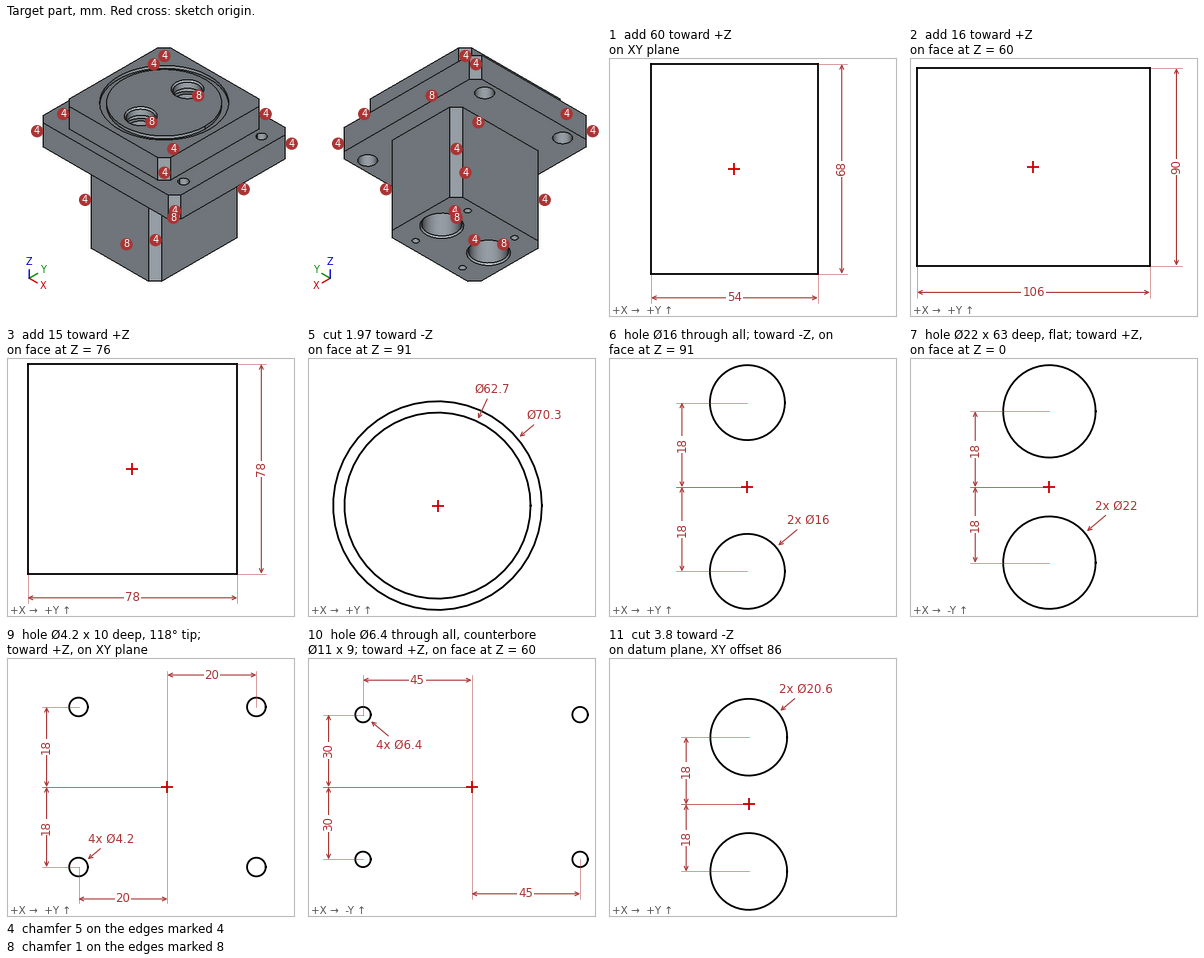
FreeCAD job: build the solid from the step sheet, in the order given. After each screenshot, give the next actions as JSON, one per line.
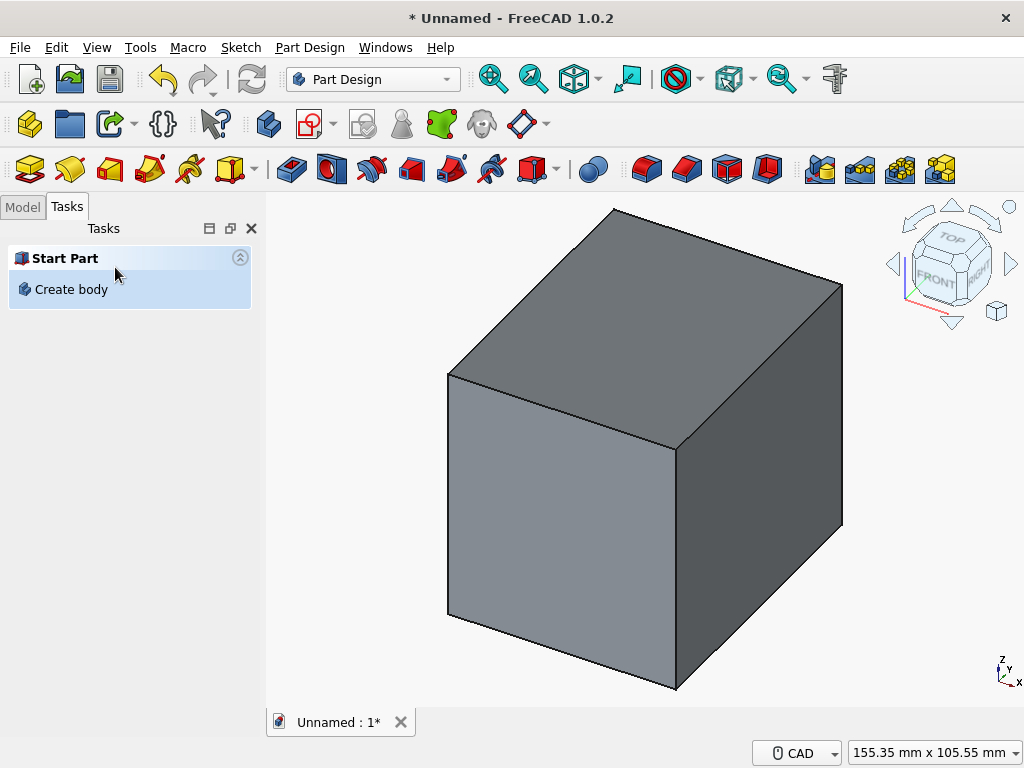
{"action": "left_click", "coordinate": [645, 329]}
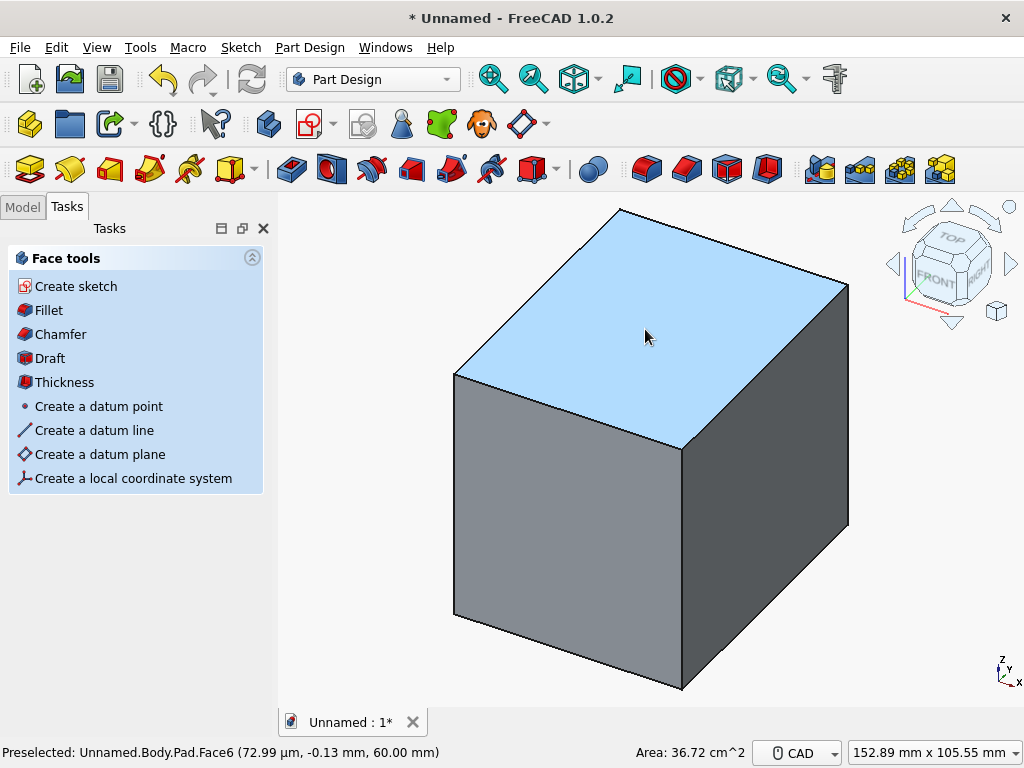
{"action": "left_click", "coordinate": [310, 124]}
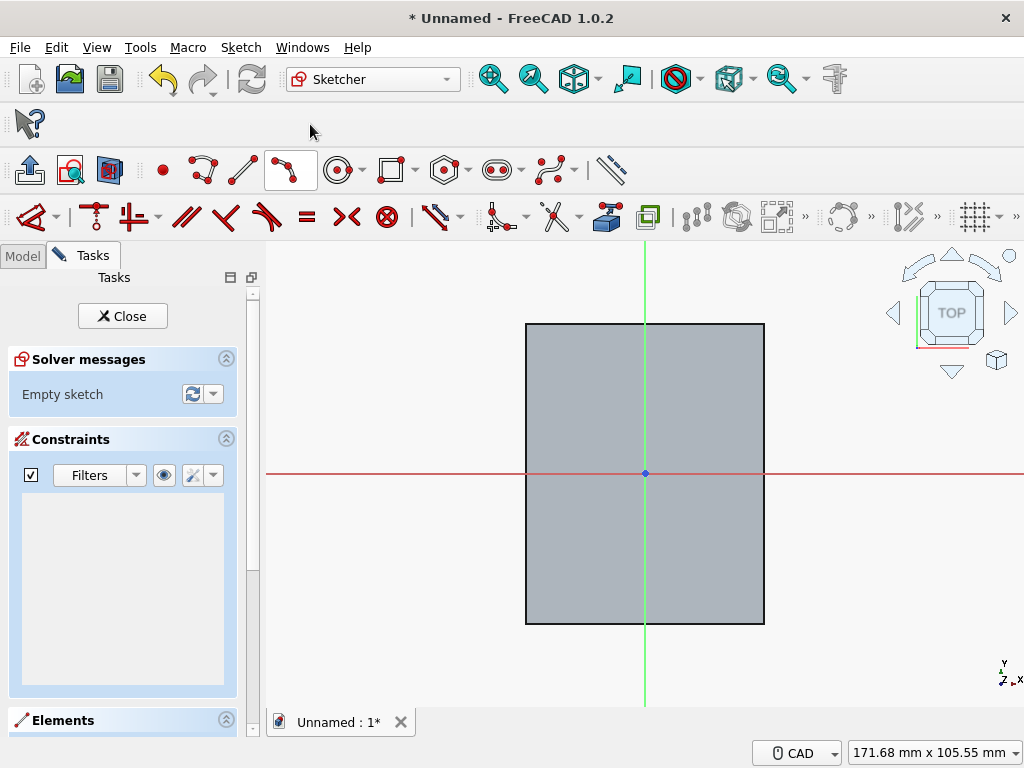
{"action": "scroll", "coordinate": [437, 474], "scroll_direction": "down", "scroll_amount": 2}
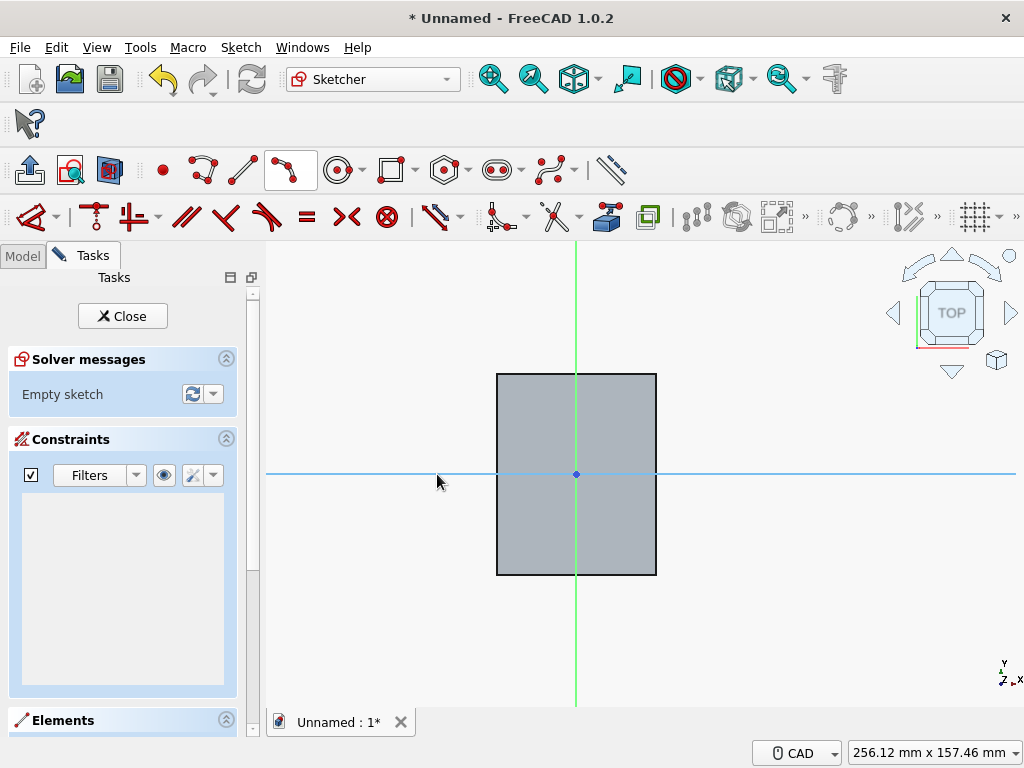
{"action": "key", "text": "g v"}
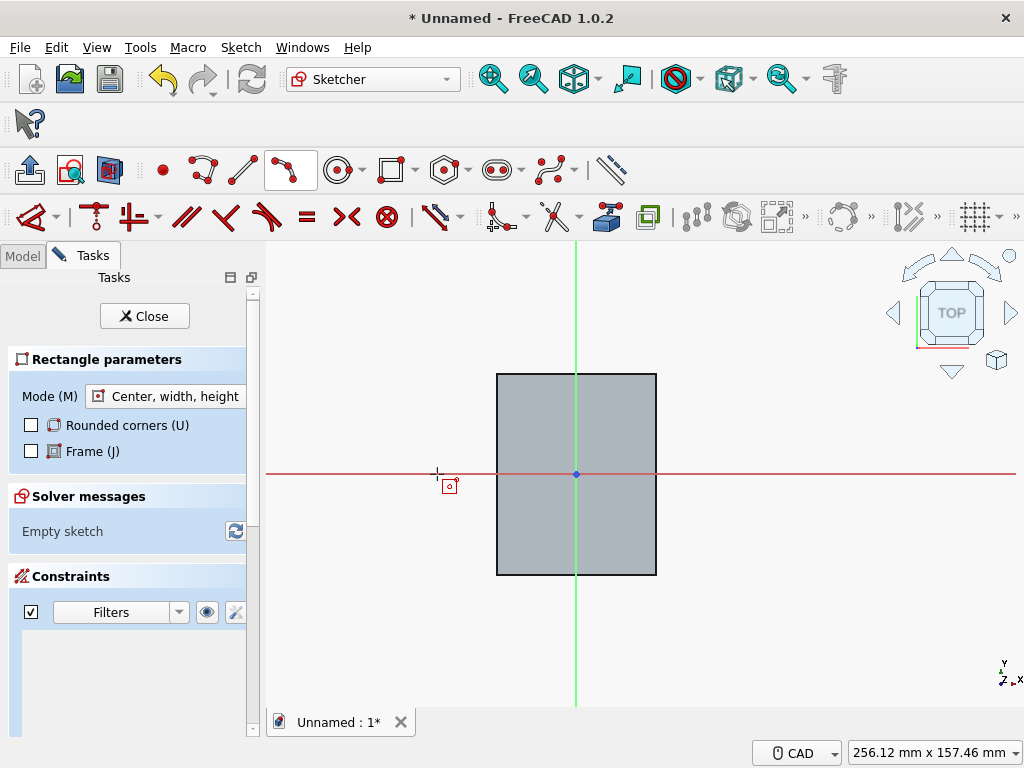
{"action": "left_click", "coordinate": [577, 474]}
{"action": "mouse_move", "coordinate": [733, 341]}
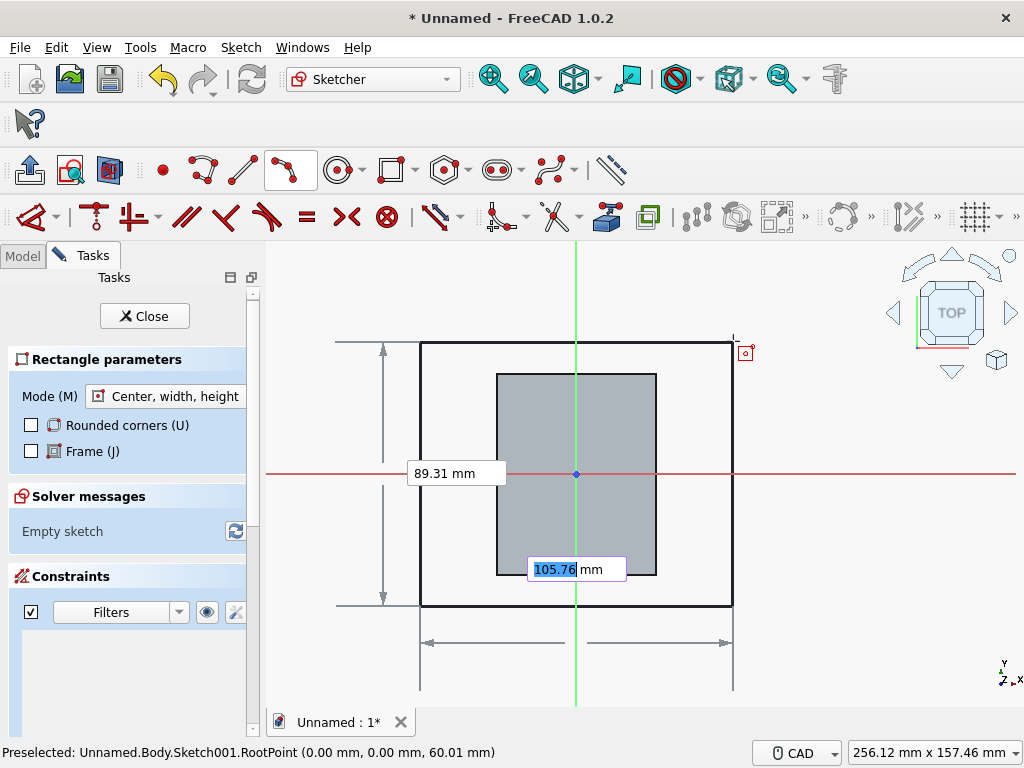
{"action": "type", "text": "106"}
{"action": "key", "text": "Tab"}
{"action": "type", "text": "90"}
{"action": "key", "text": "Return"}
{"action": "key", "text": "Escape"}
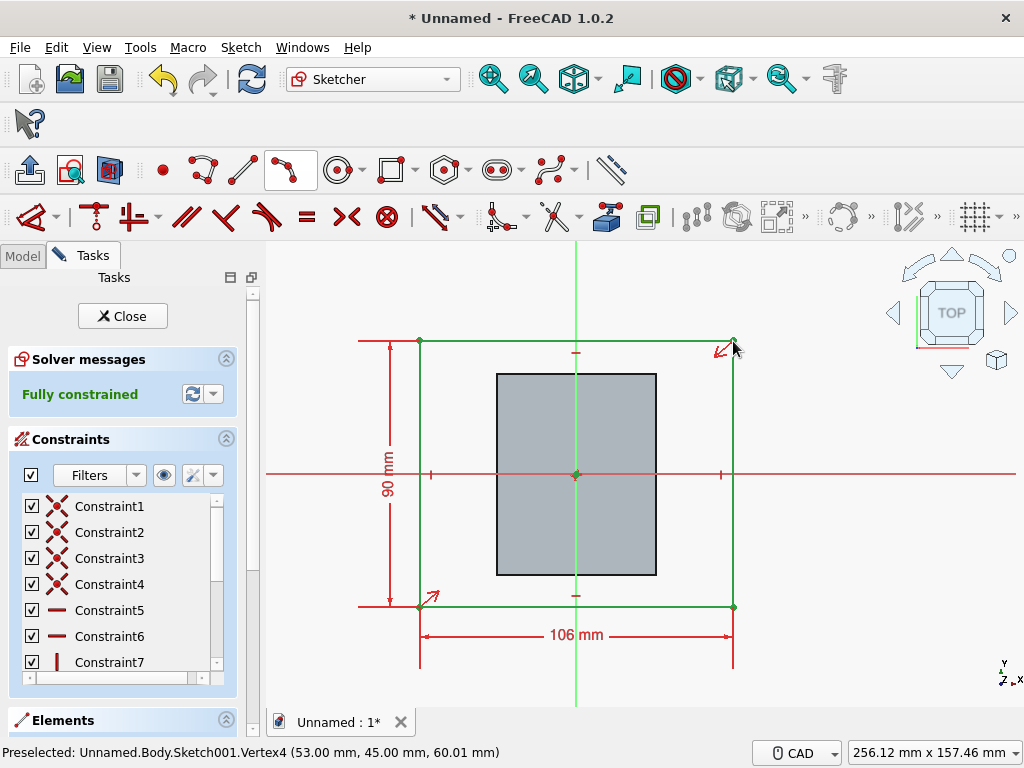
{"action": "left_click", "coordinate": [123, 316]}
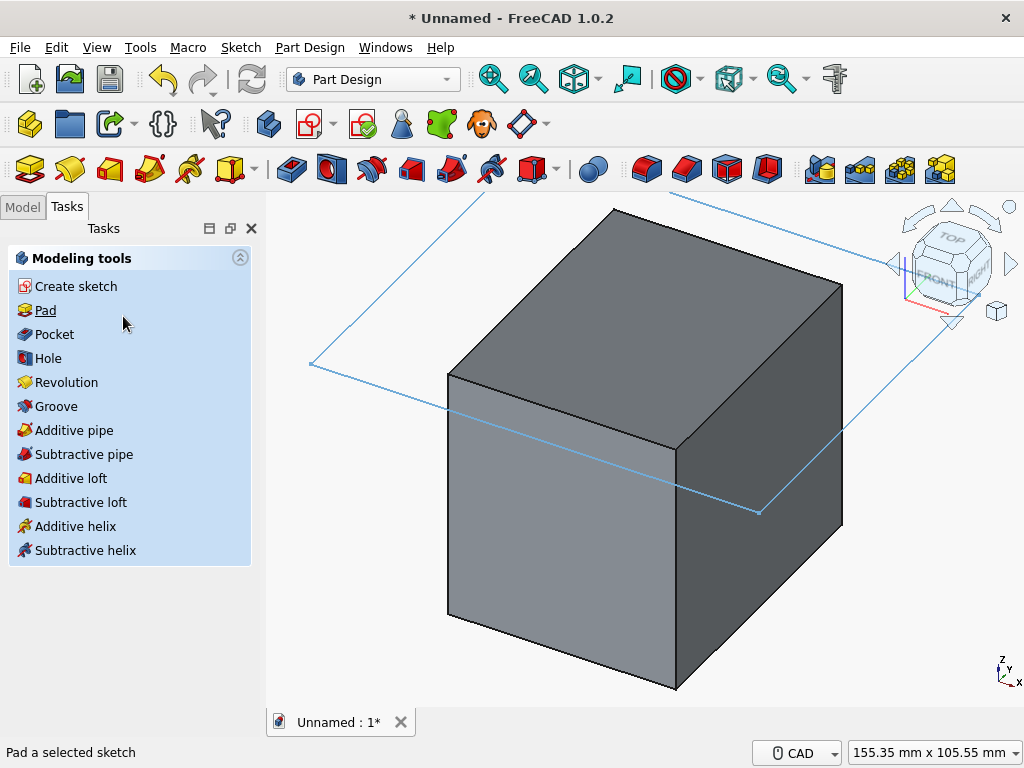
{"action": "left_click", "coordinate": [30, 170]}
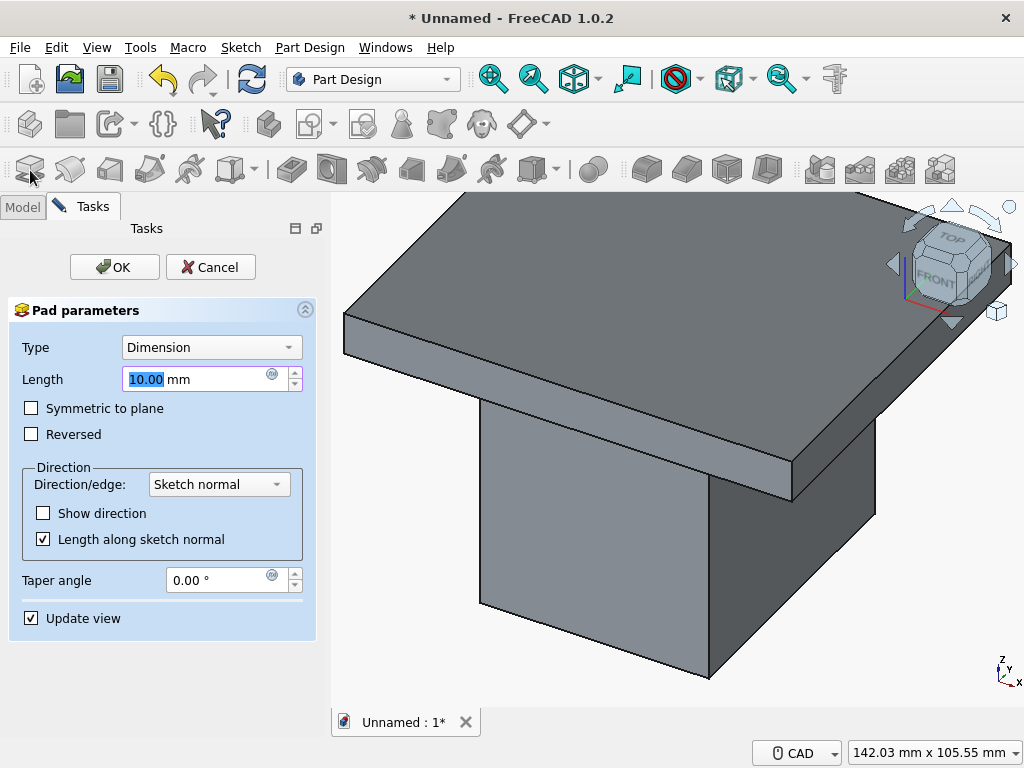
{"action": "type", "text": "16"}
{"action": "key", "text": "Tab"}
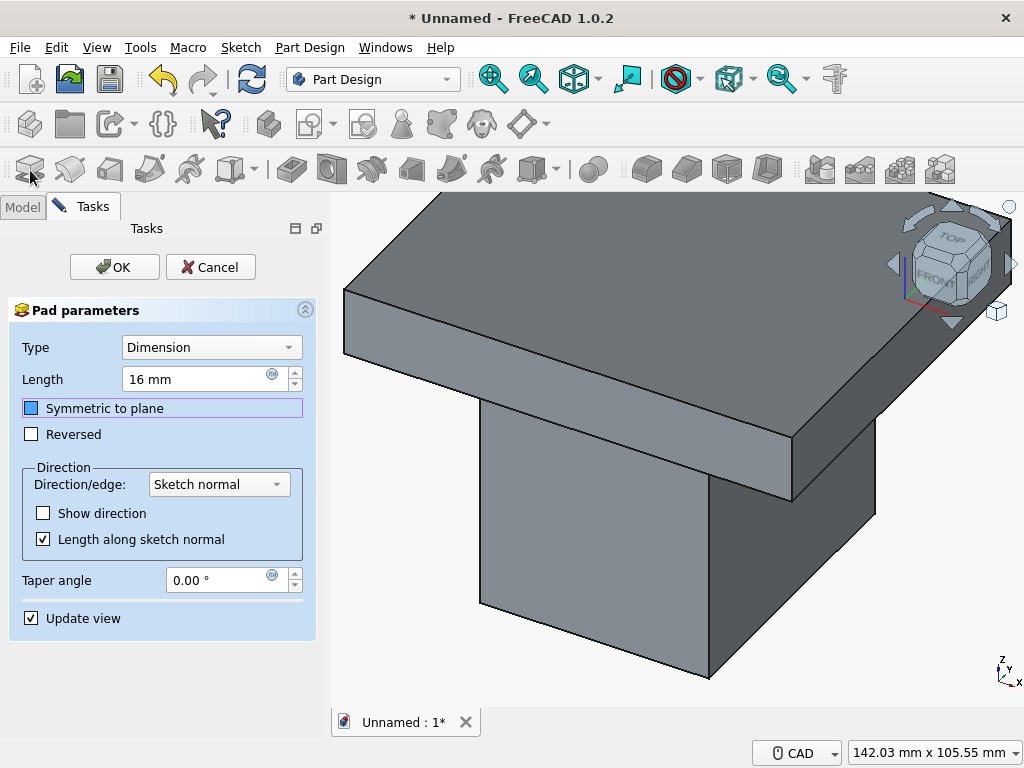
{"action": "left_click", "coordinate": [115, 267]}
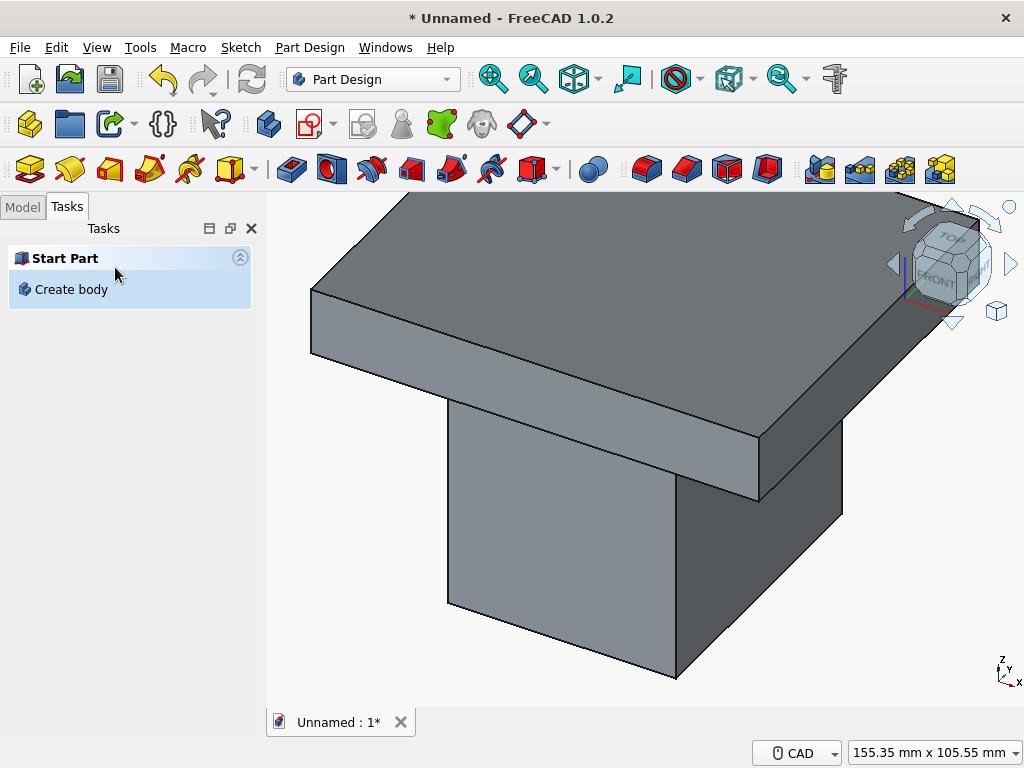
{"action": "key", "text": "v f"}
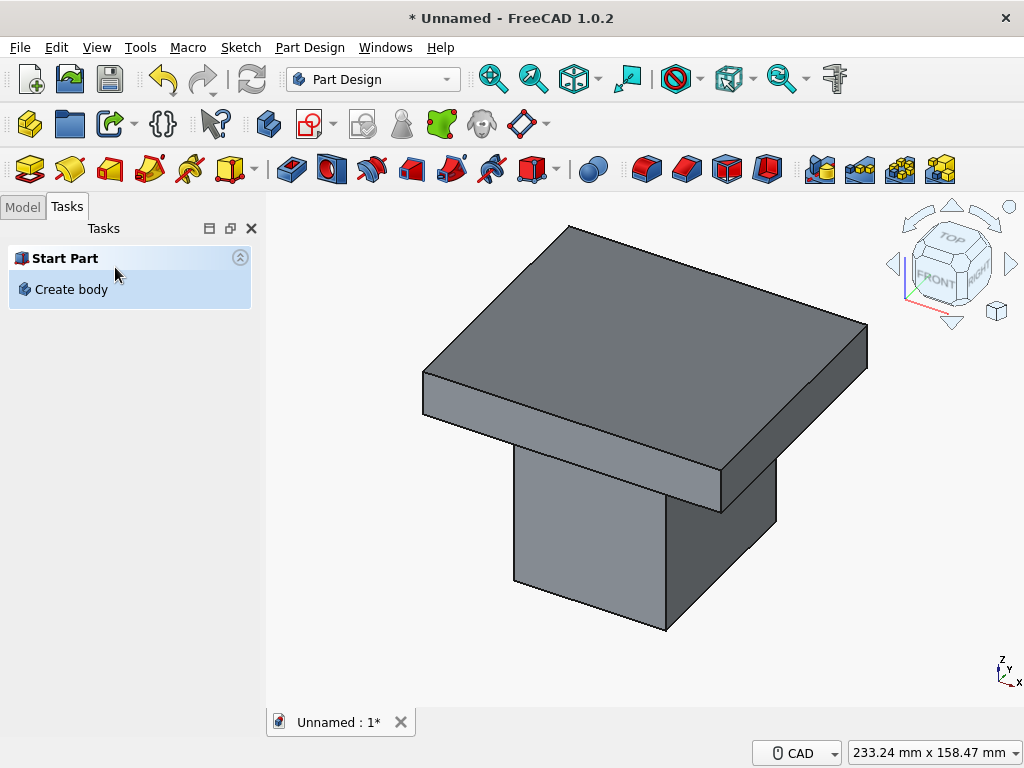
{"action": "left_click", "coordinate": [645, 347]}